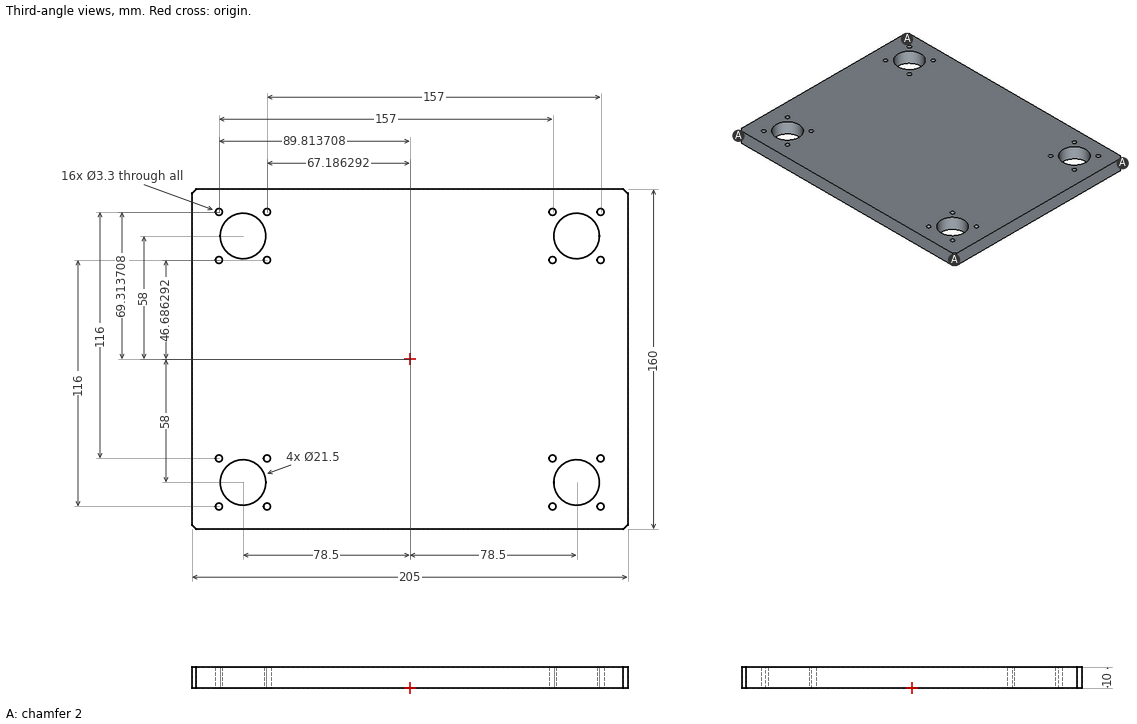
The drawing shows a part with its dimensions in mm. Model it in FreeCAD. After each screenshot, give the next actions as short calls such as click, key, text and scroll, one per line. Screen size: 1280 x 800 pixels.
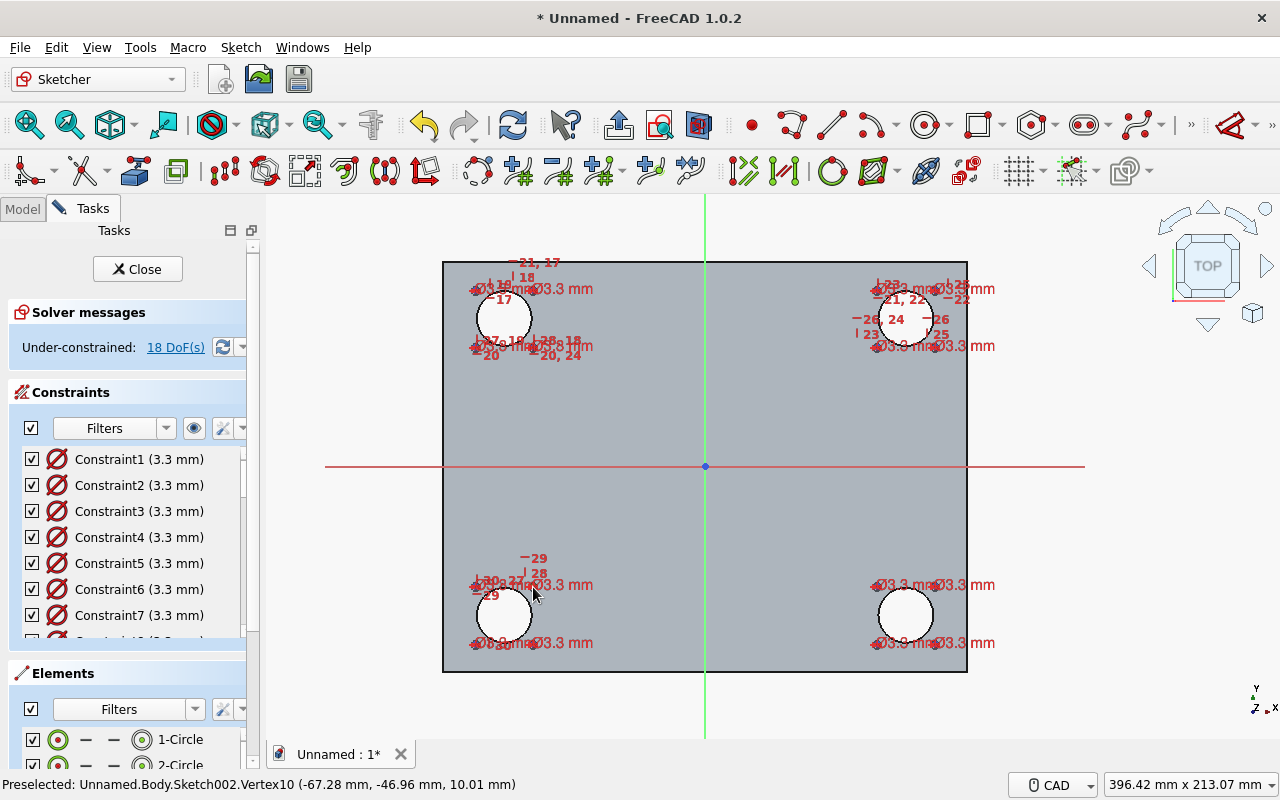
click(533, 645)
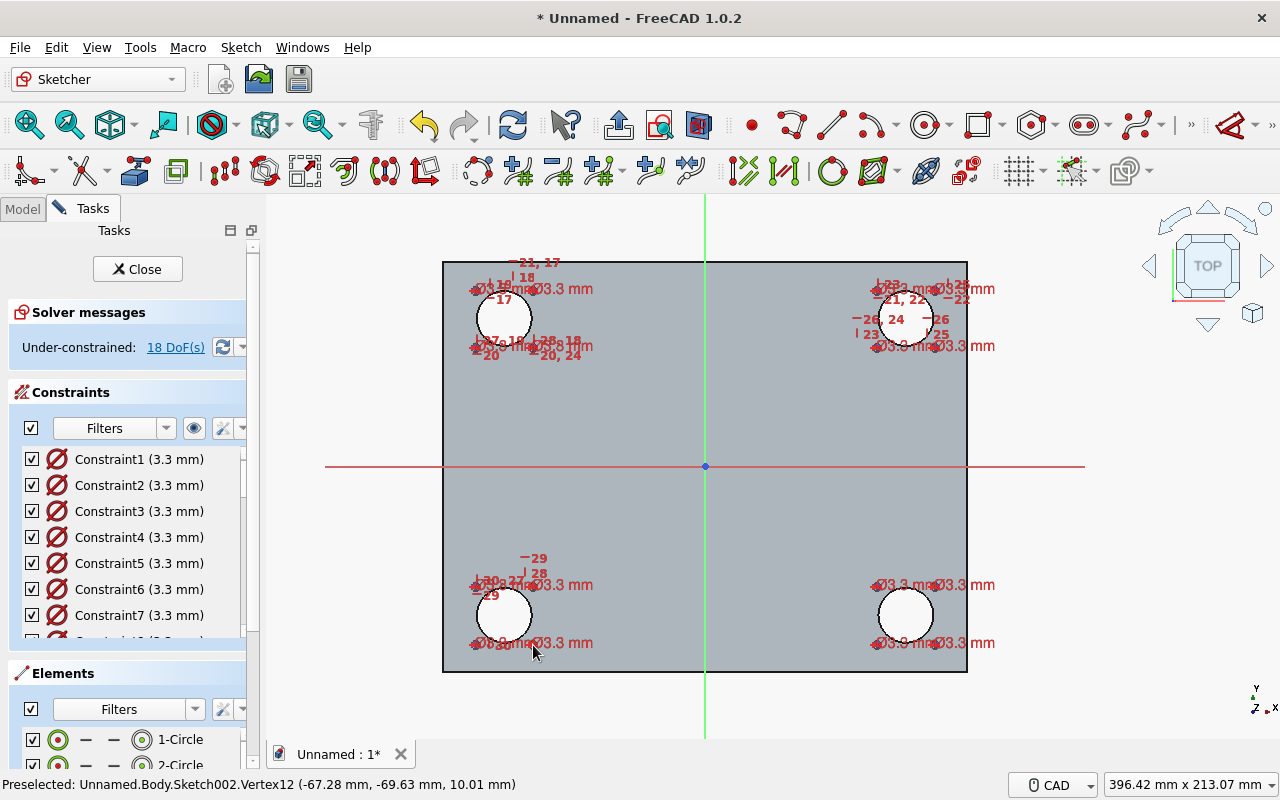
key(v)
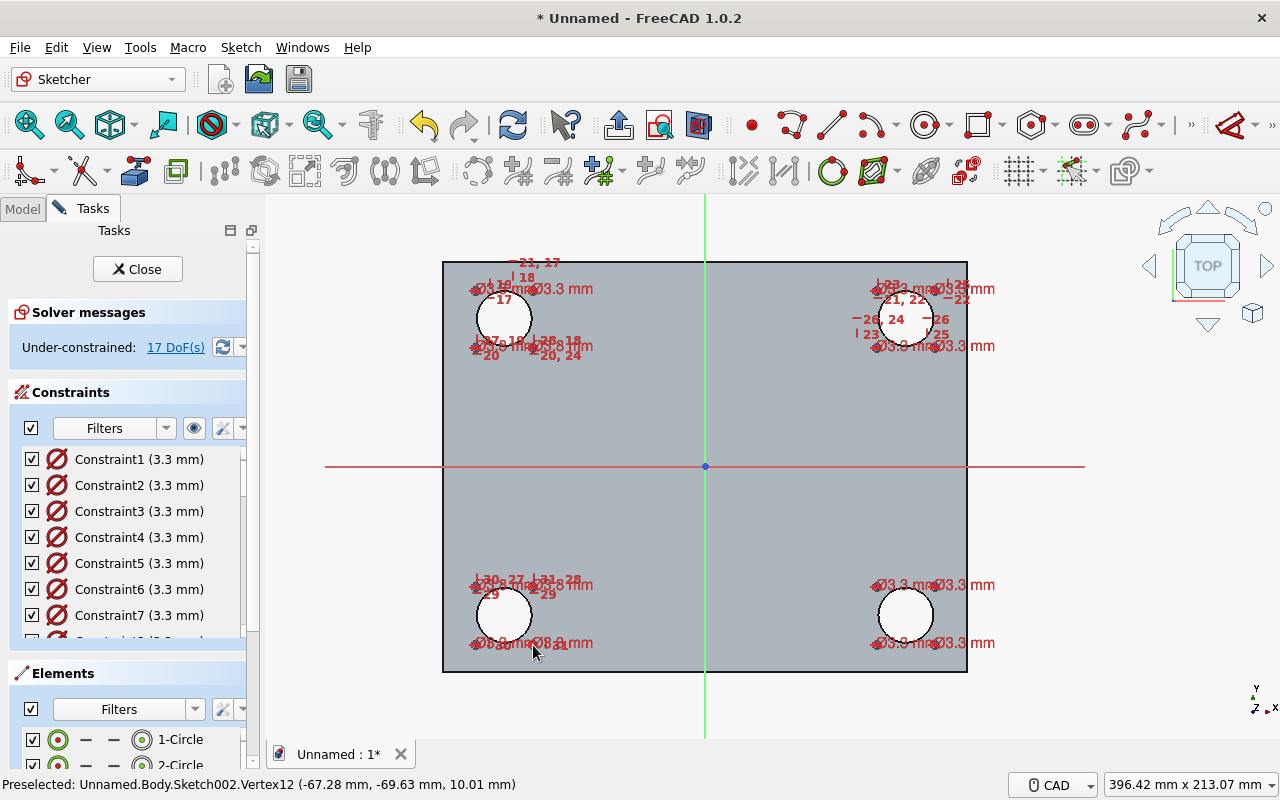
click(476, 645)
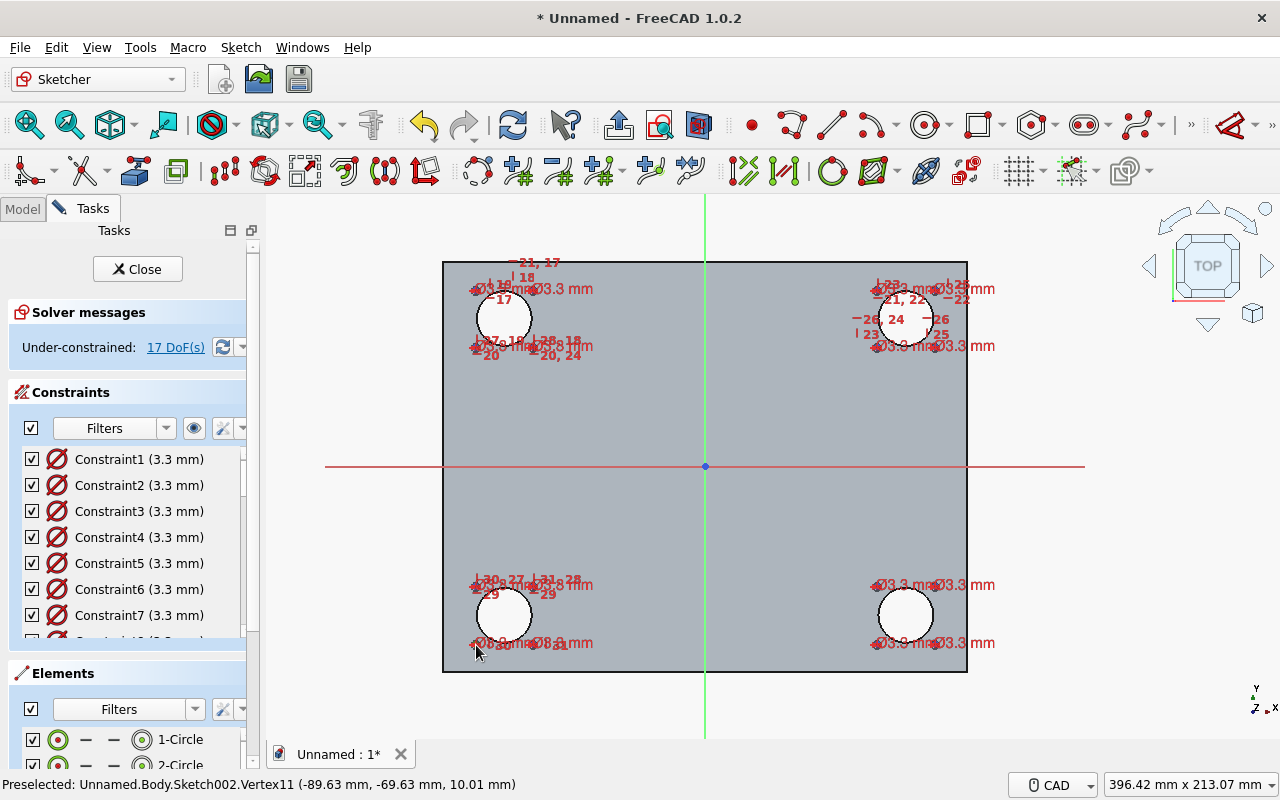
click(533, 645)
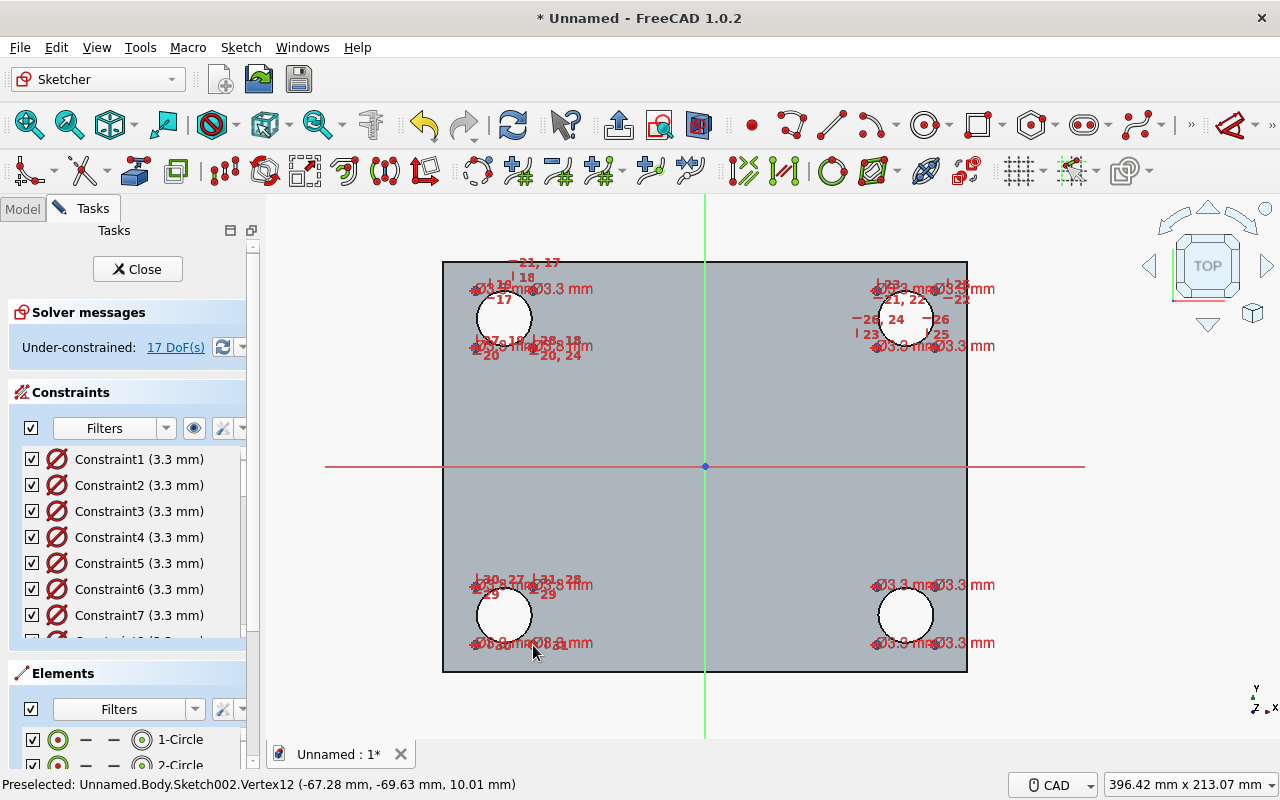
key(h)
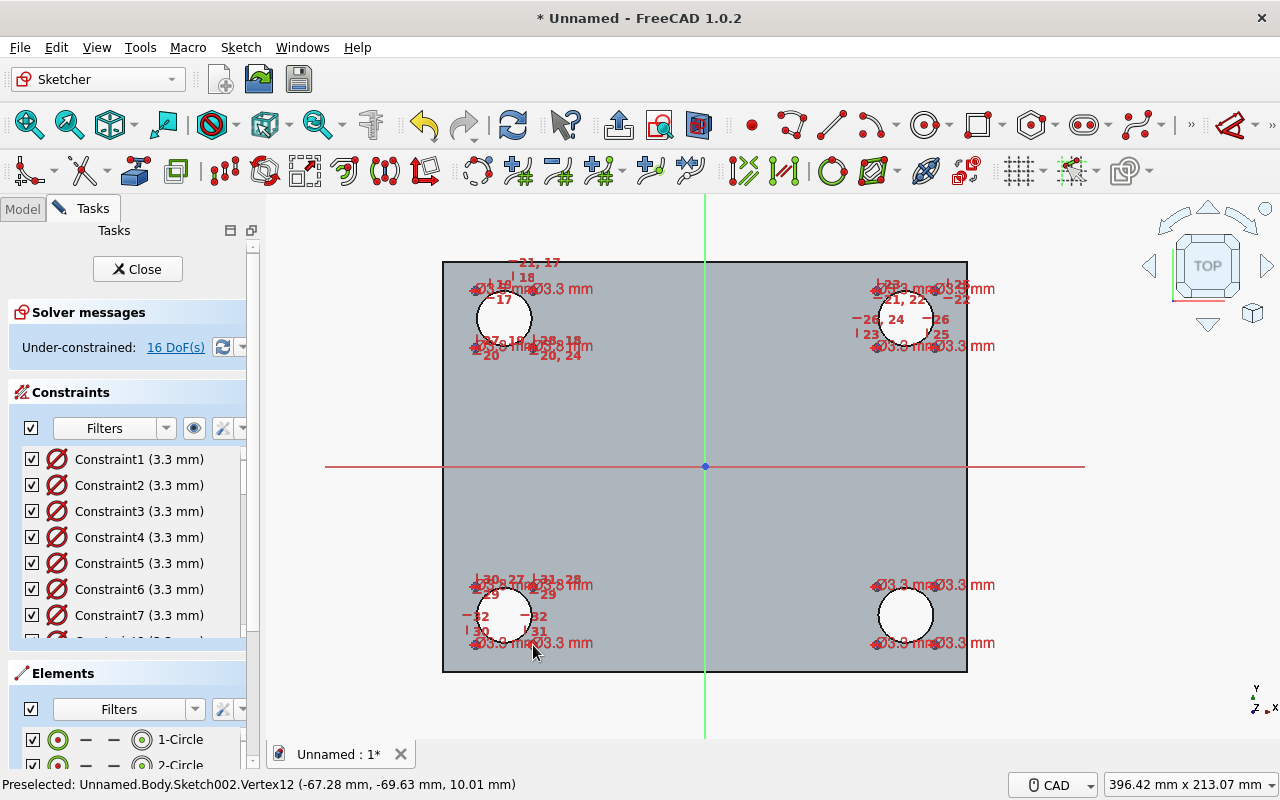
click(877, 348)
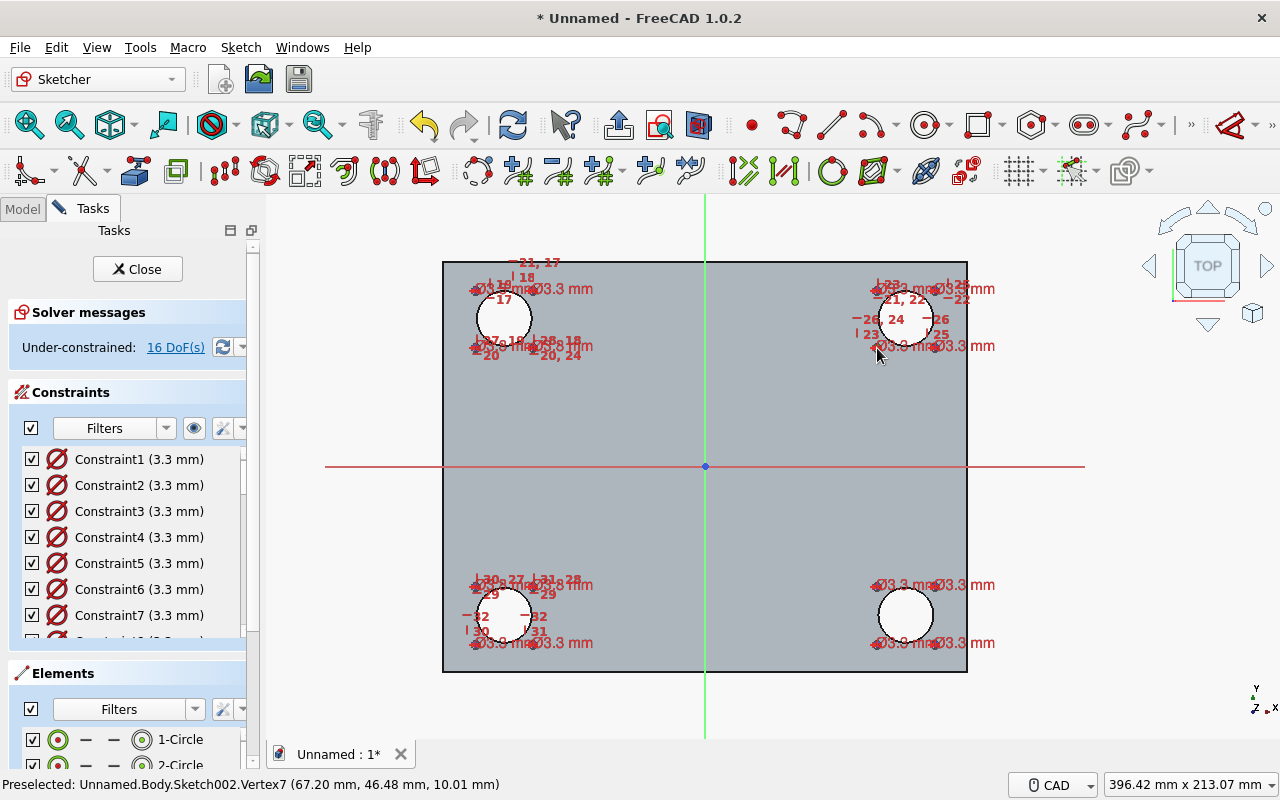
click(877, 587)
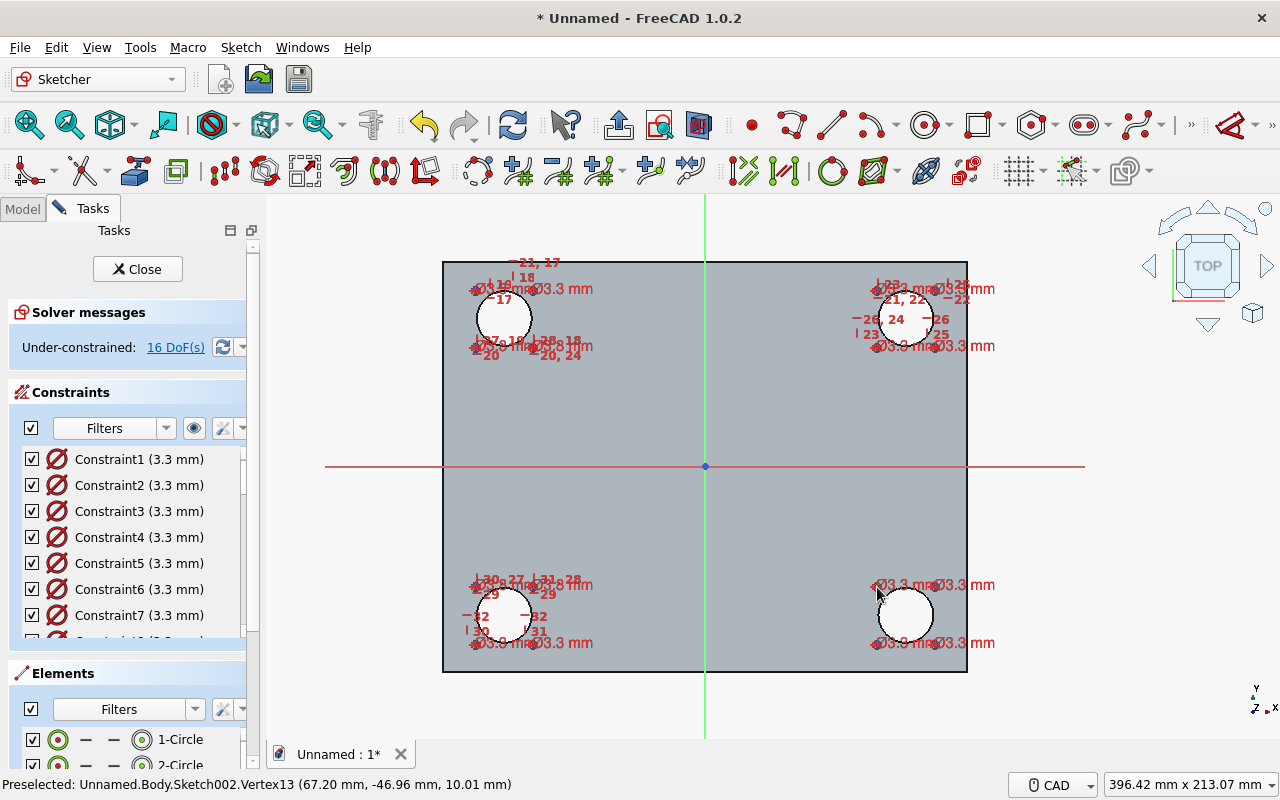
key(v)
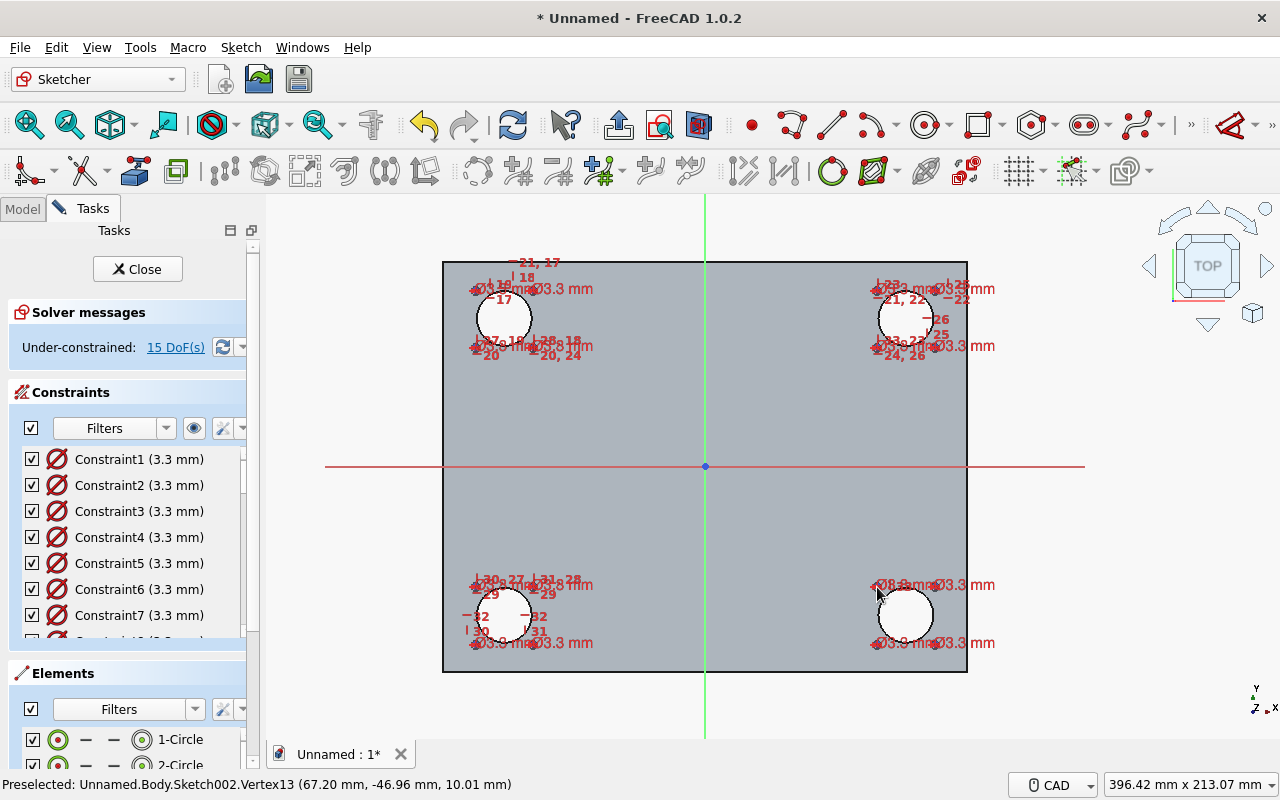
click(533, 587)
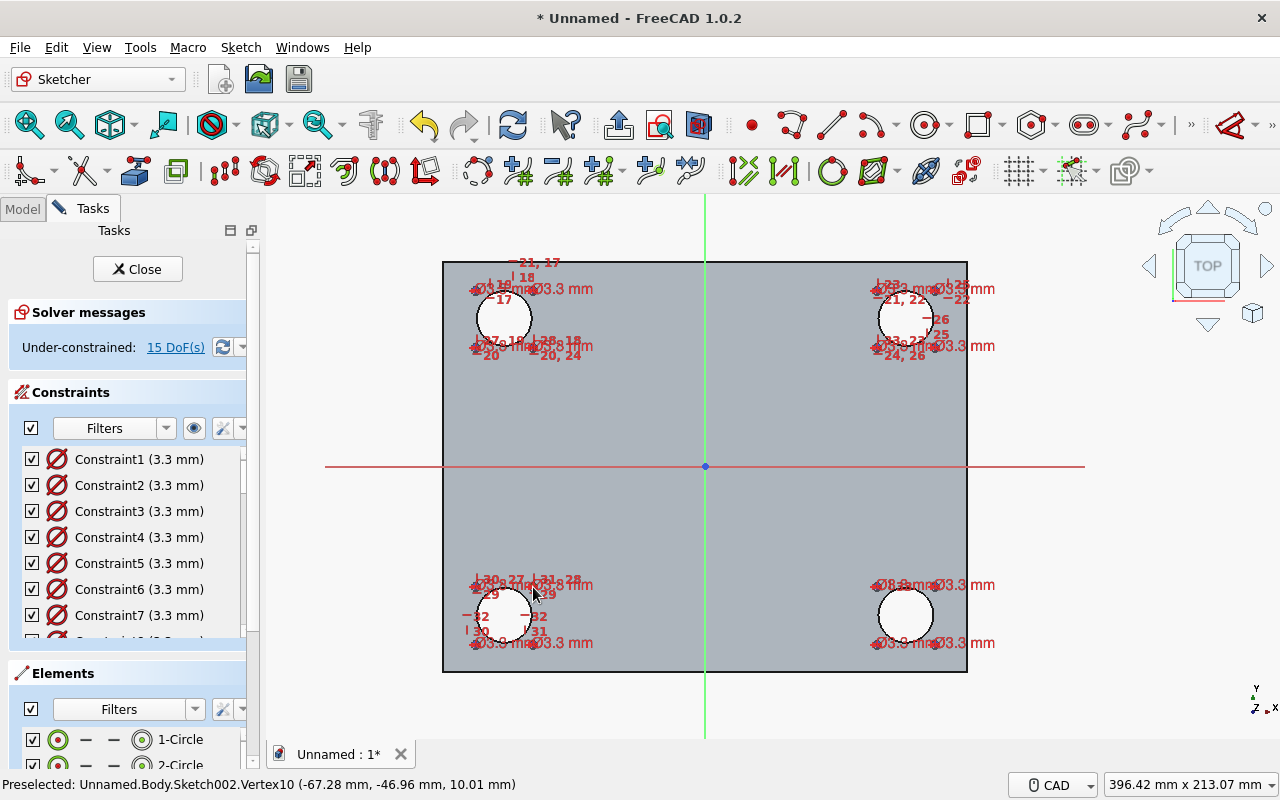
click(877, 587)